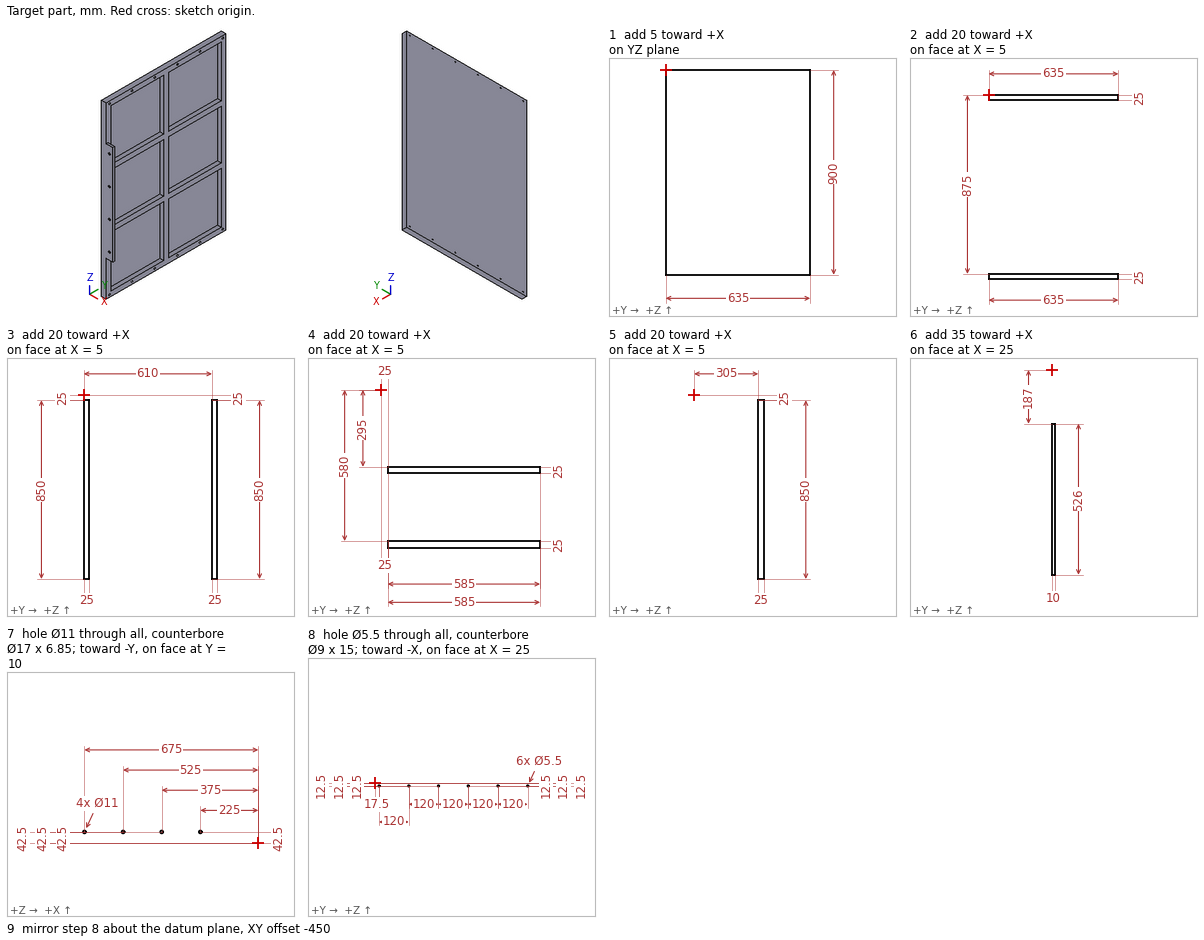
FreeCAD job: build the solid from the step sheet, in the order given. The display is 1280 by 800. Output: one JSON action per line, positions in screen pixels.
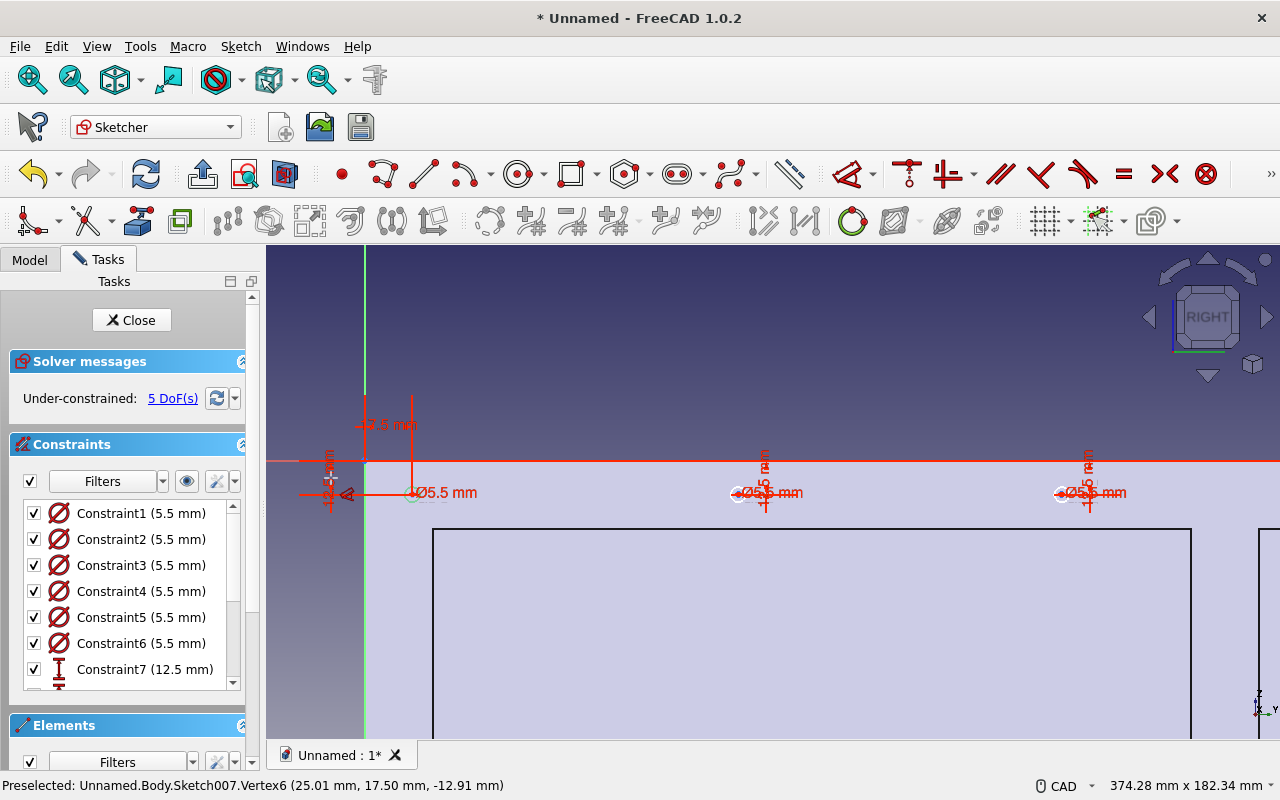
{"action": "scroll", "coordinate": [413, 498], "scroll_direction": "down", "scroll_amount": 5}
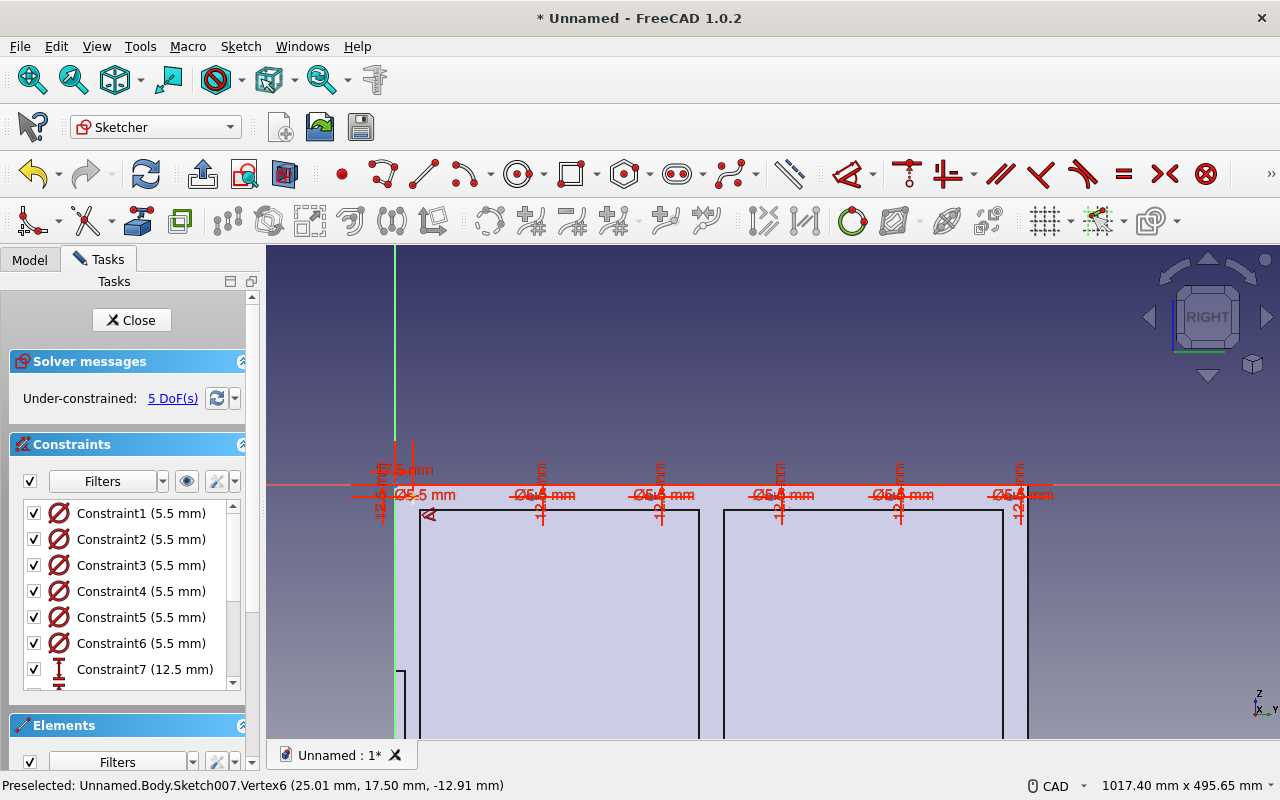
{"action": "left_click", "coordinate": [1011, 497]}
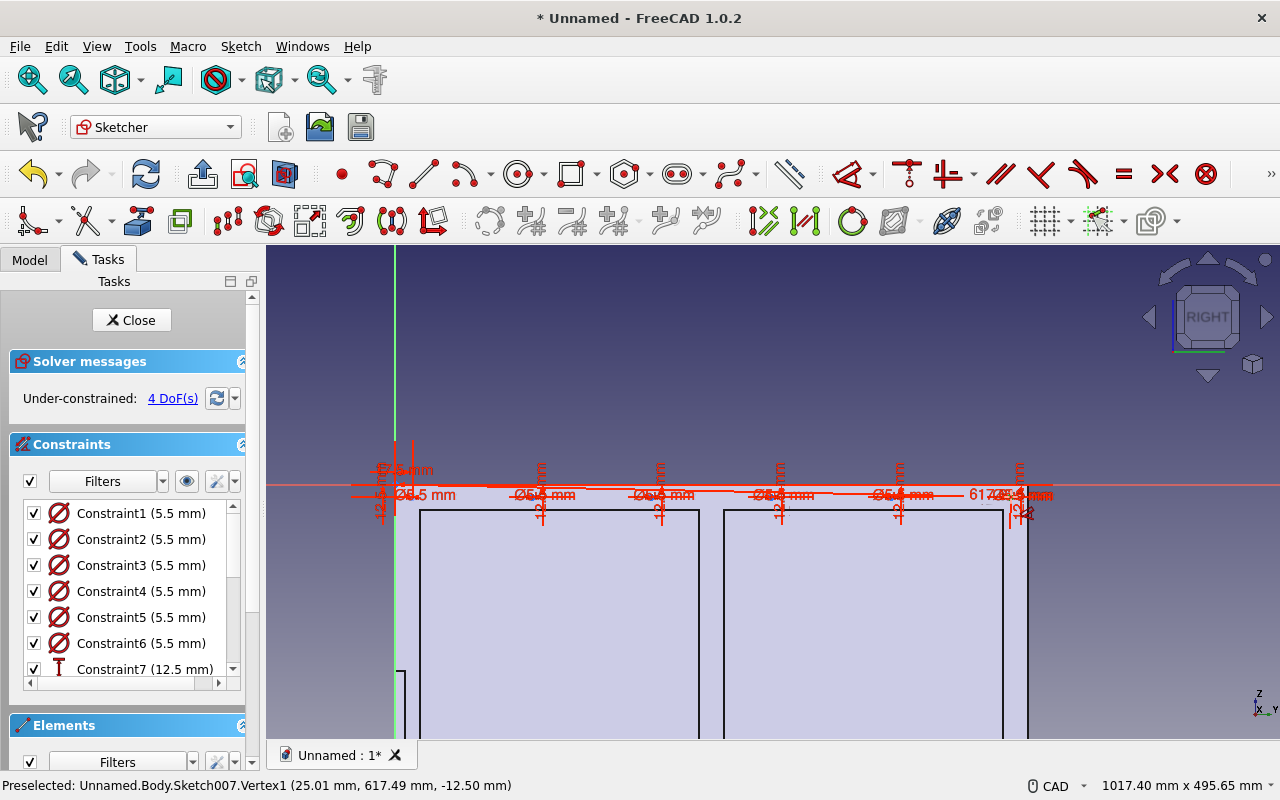
{"action": "left_click", "coordinate": [891, 497]}
{"action": "left_click", "coordinate": [951, 531]}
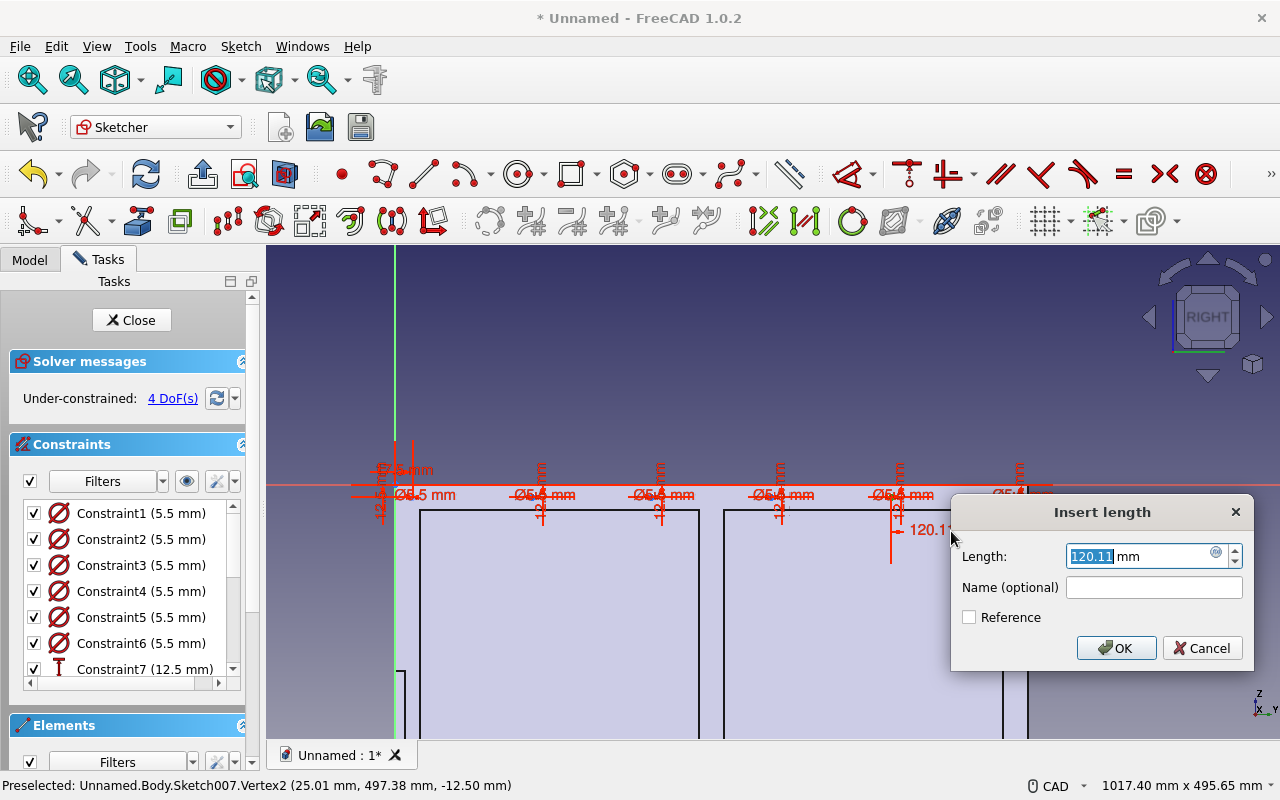
{"action": "type", "text": "120"}
{"action": "key", "text": "Return"}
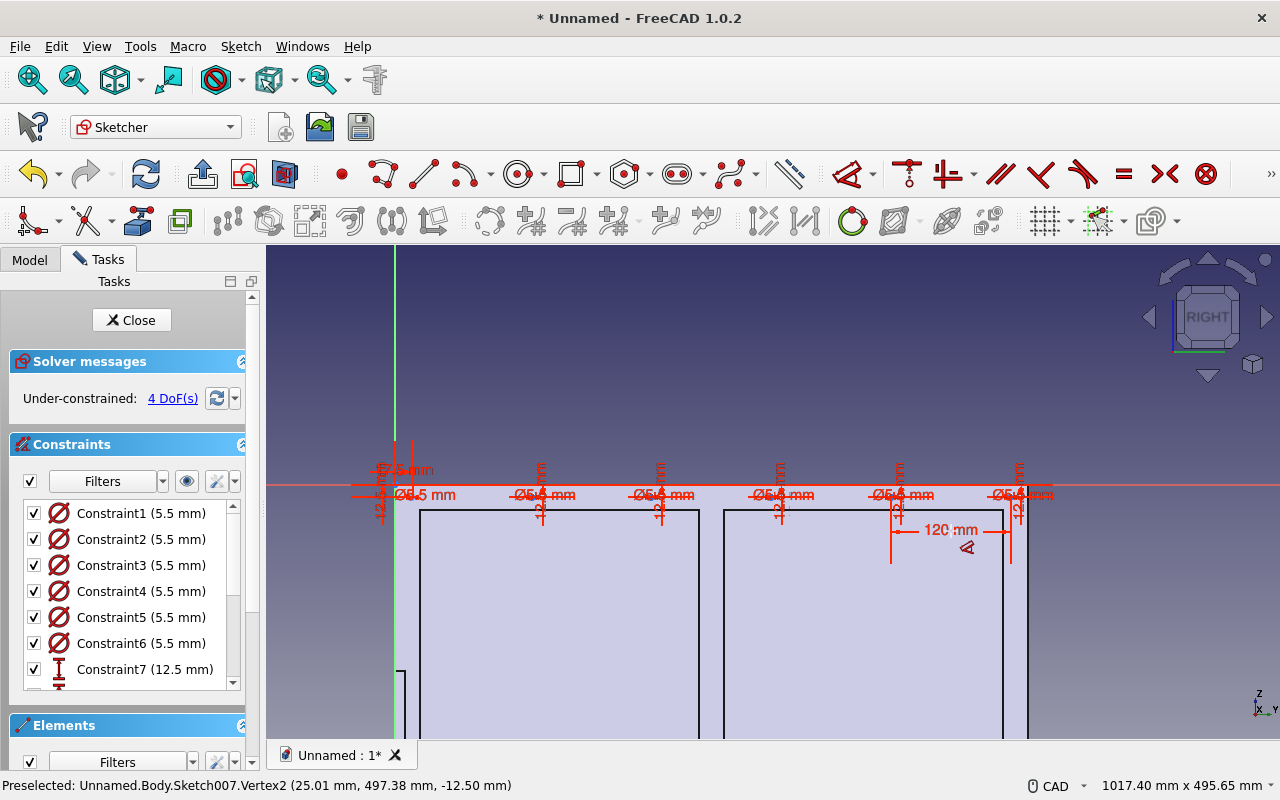
{"action": "left_click", "coordinate": [891, 497]}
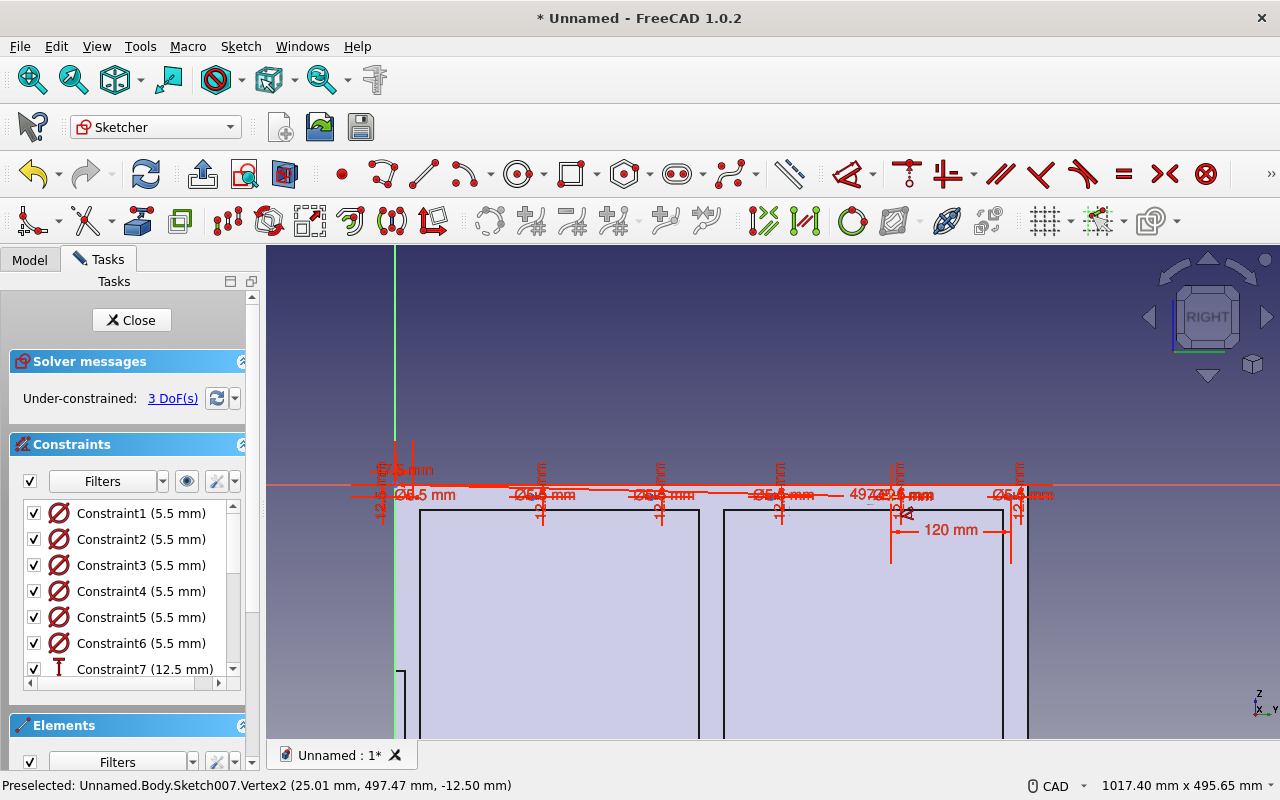
{"action": "left_click", "coordinate": [771, 497]}
{"action": "left_click", "coordinate": [831, 531]}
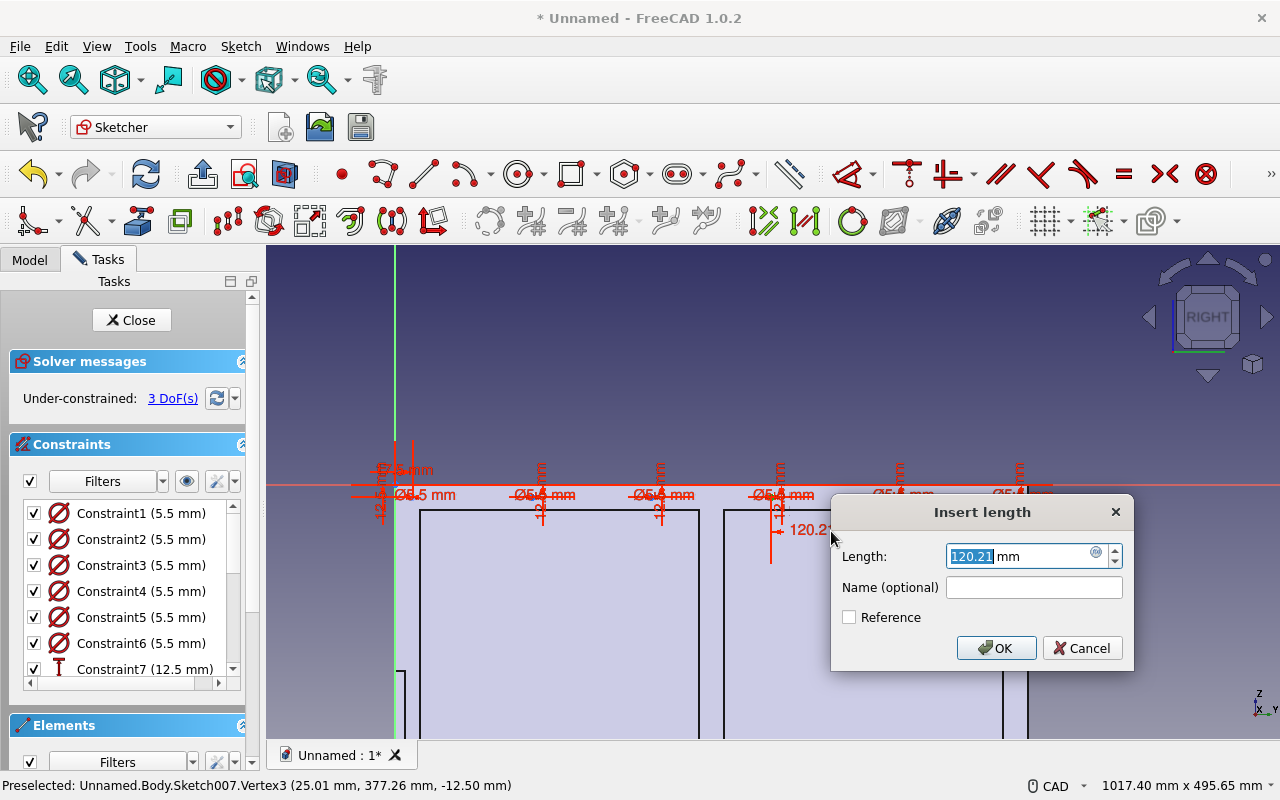
{"action": "type", "text": "120"}
{"action": "key", "text": "Return"}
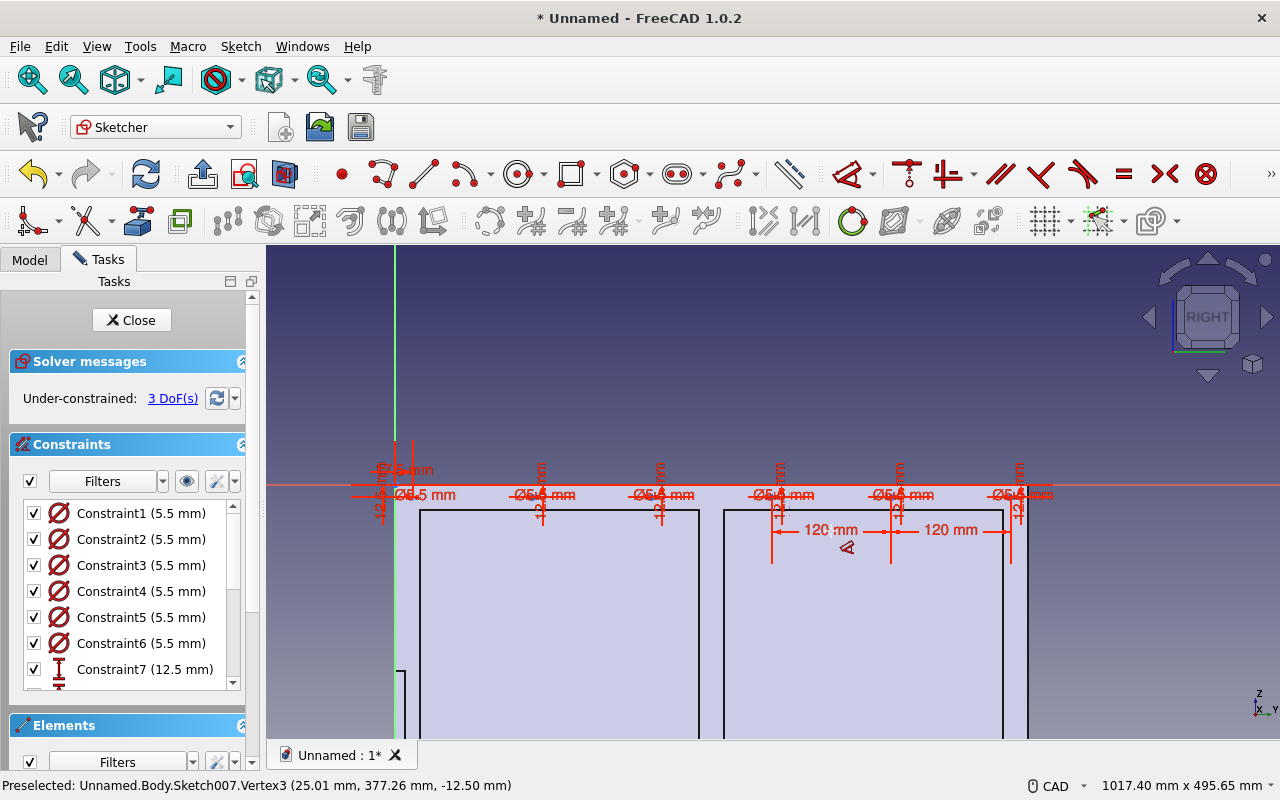
{"action": "left_click", "coordinate": [772, 497]}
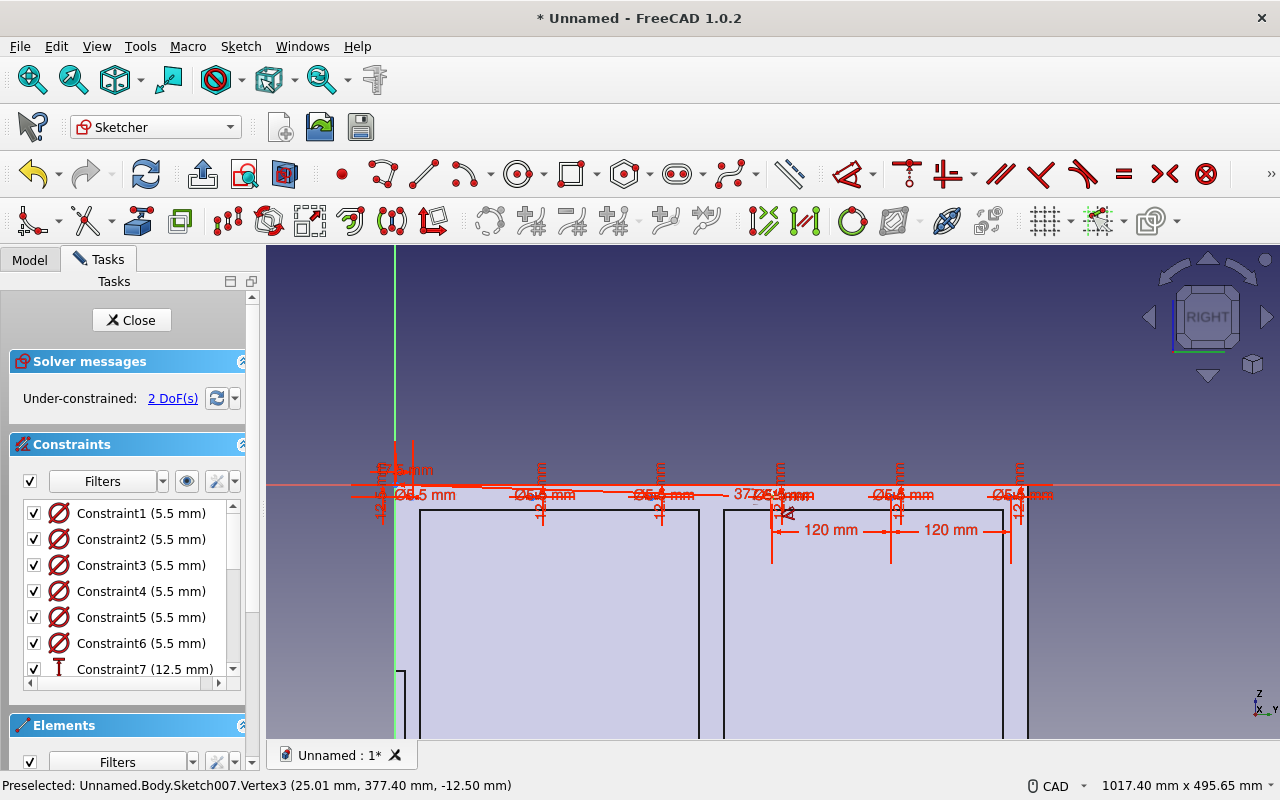
{"action": "left_click", "coordinate": [652, 497]}
{"action": "left_click", "coordinate": [712, 531]}